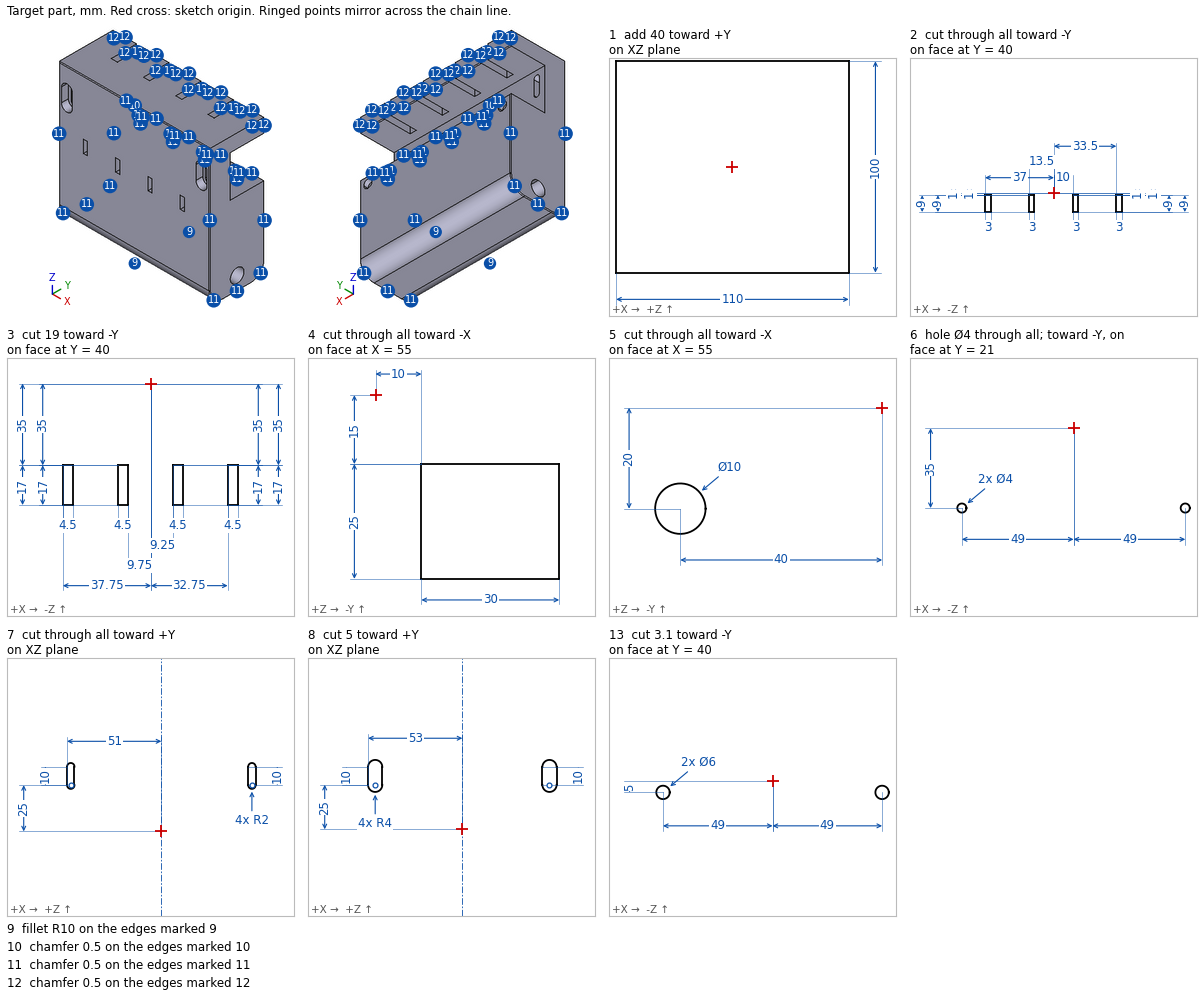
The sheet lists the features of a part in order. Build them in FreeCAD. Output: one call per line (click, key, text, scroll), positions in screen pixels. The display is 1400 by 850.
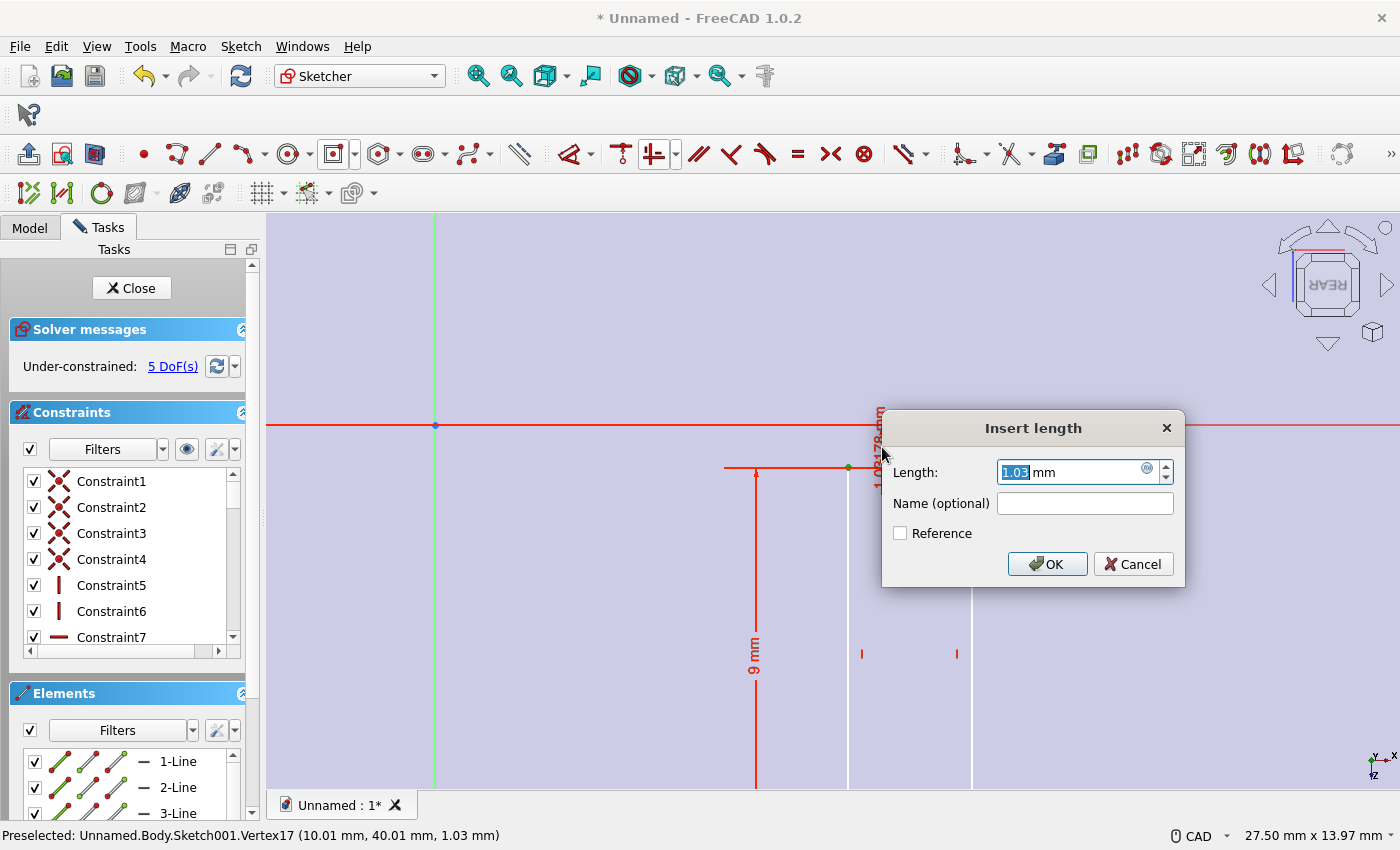
text(1)
key(Return)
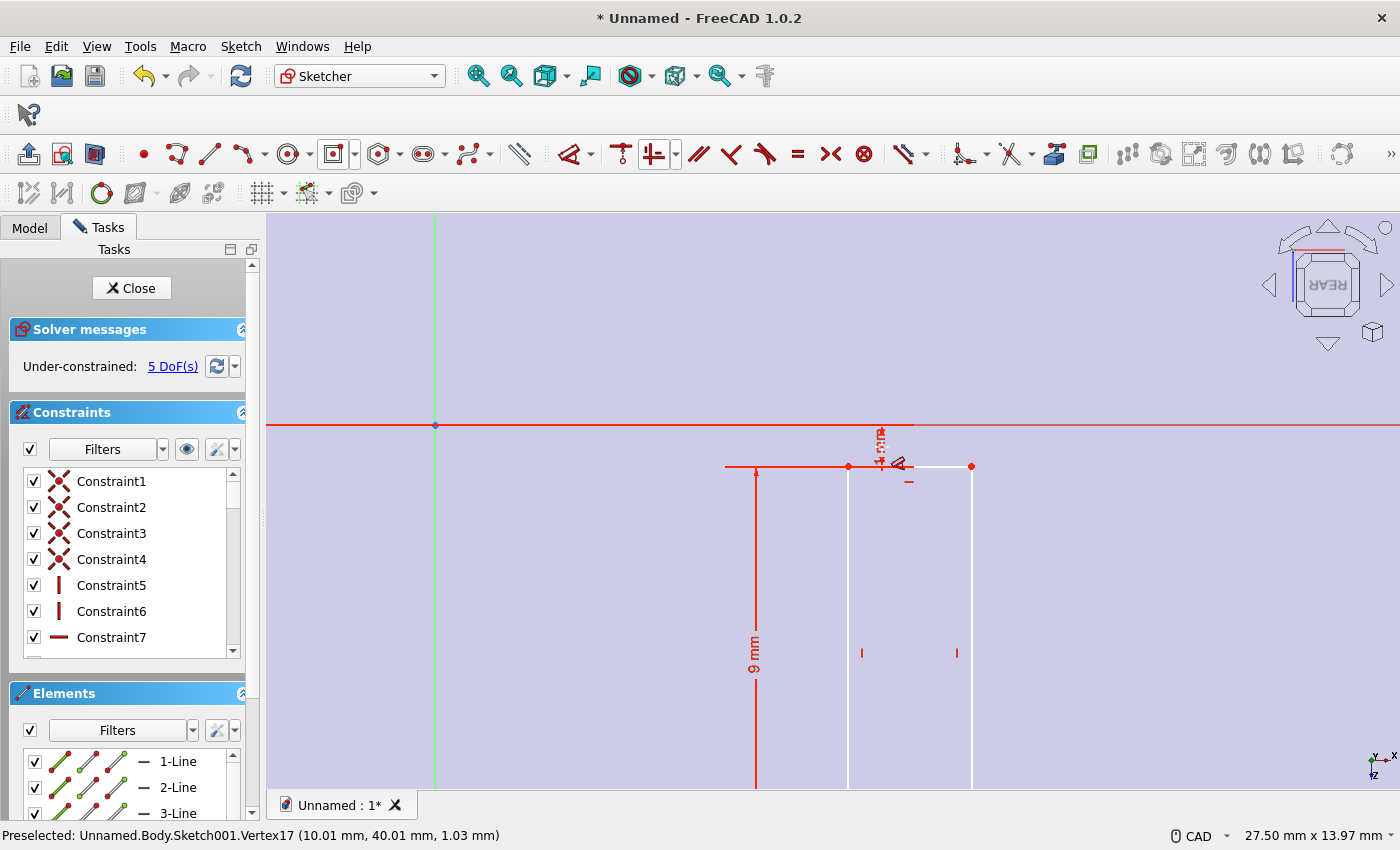
scroll(850, 468, down, 8)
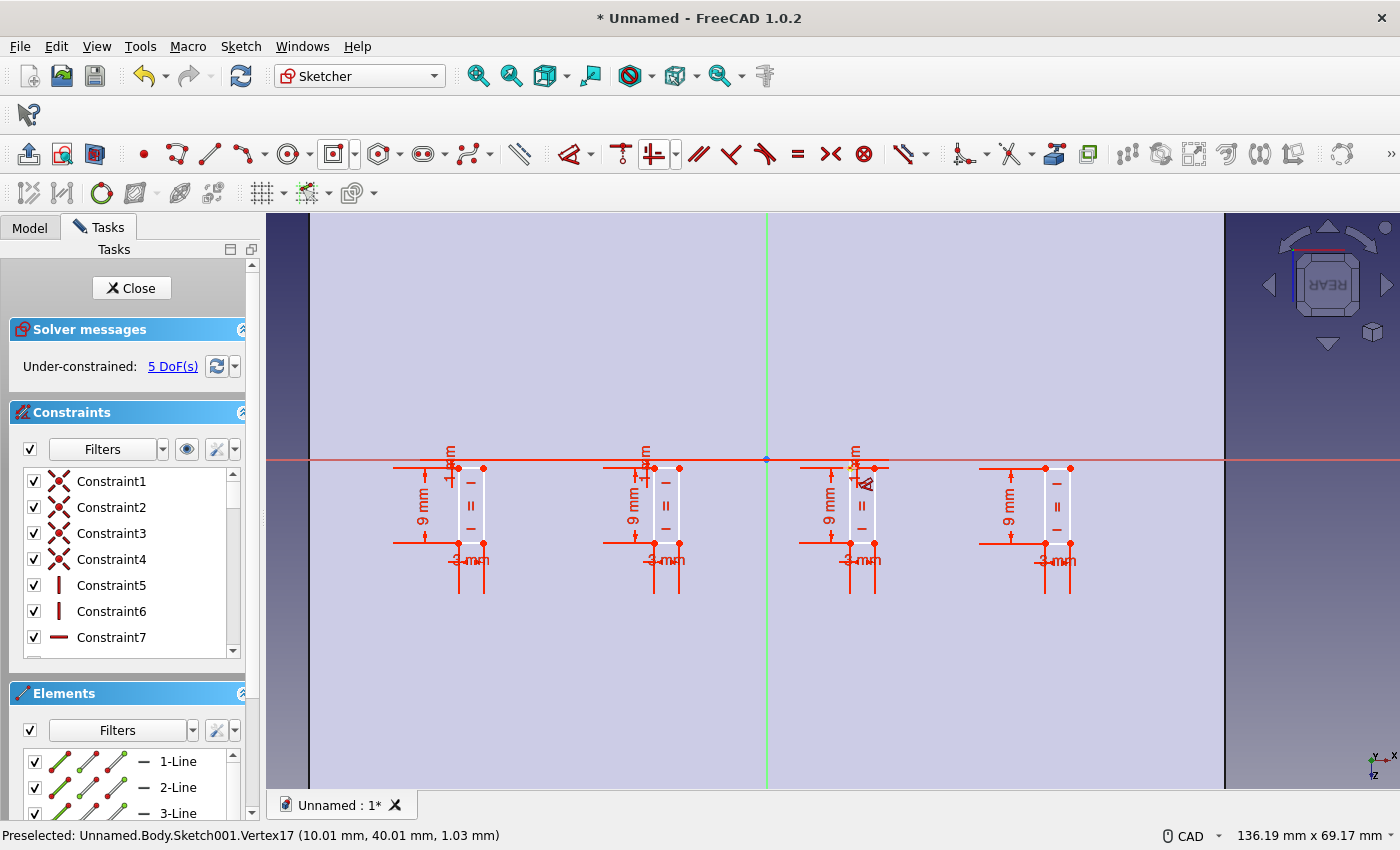
scroll(1045, 469, up, 8)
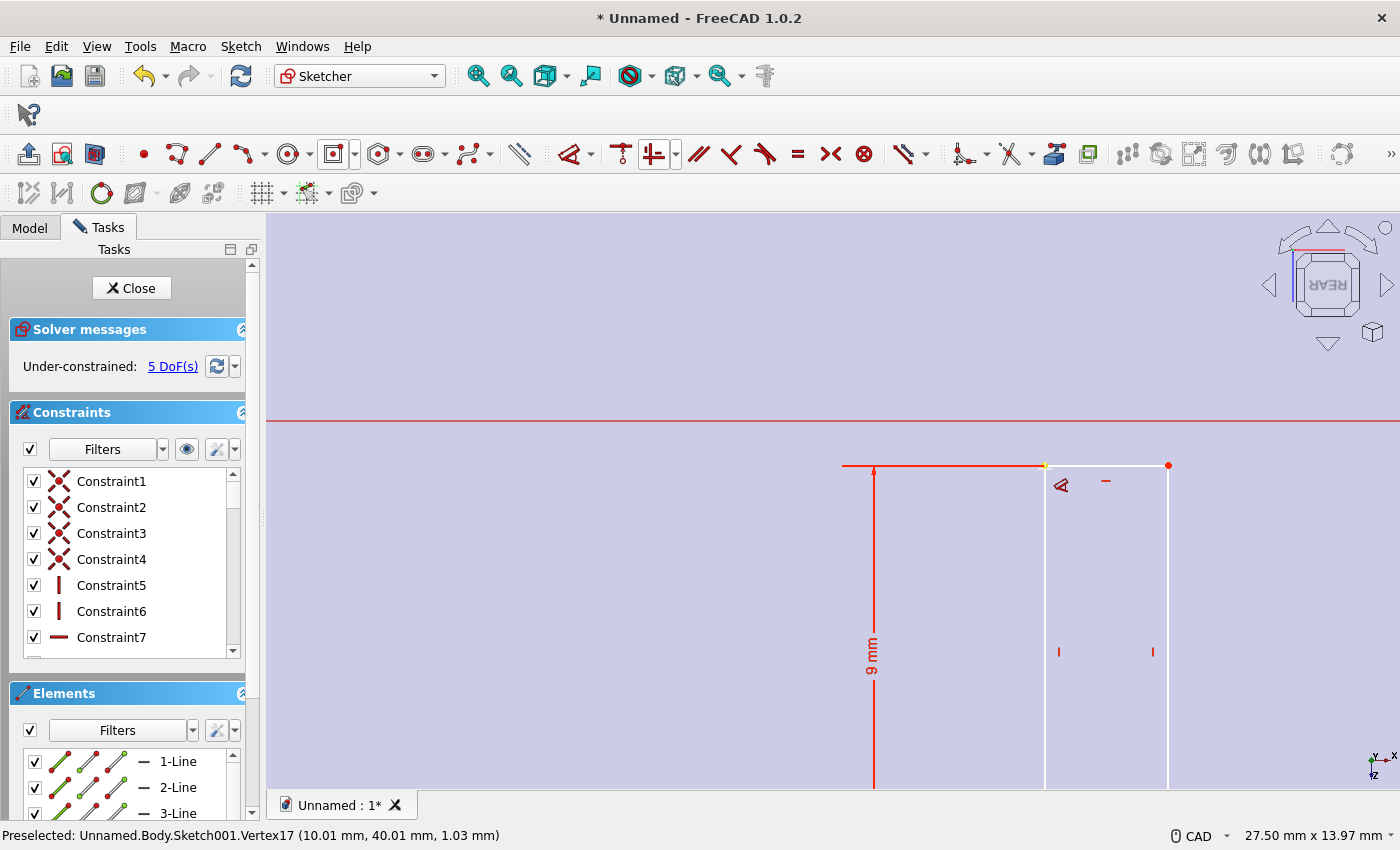
click(1045, 466)
click(1079, 444)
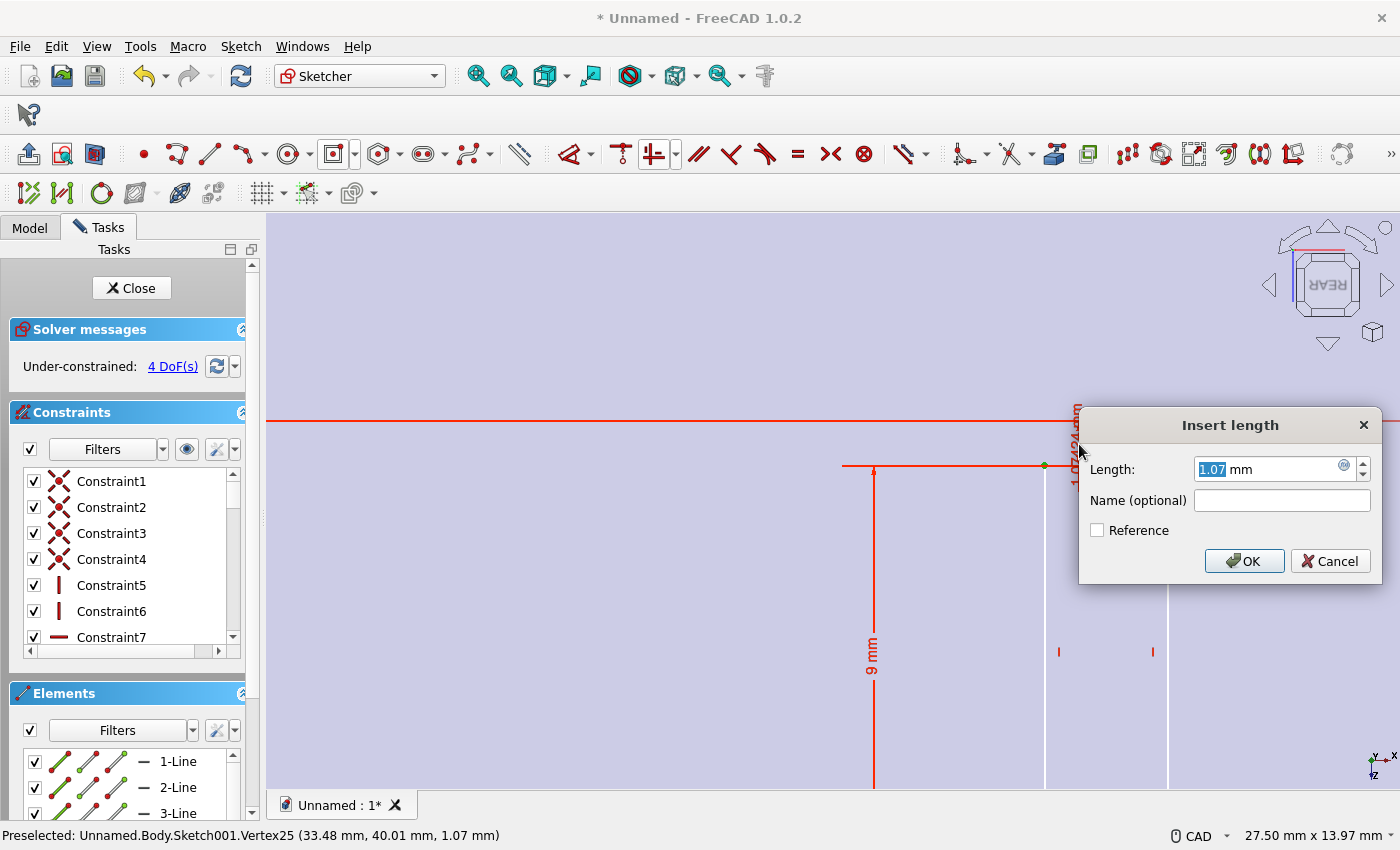
text(1)
key(Return)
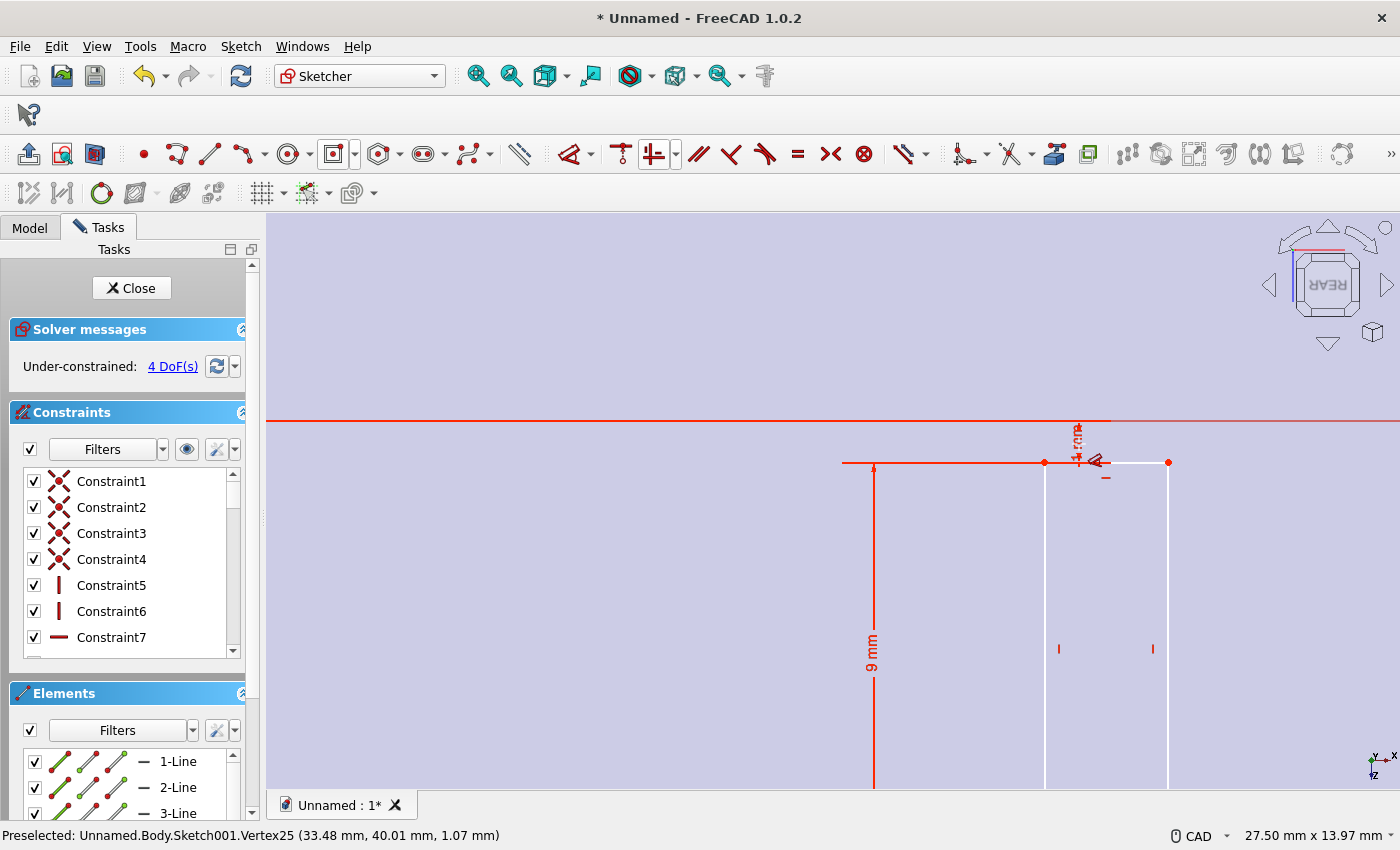
scroll(1046, 469, down, 8)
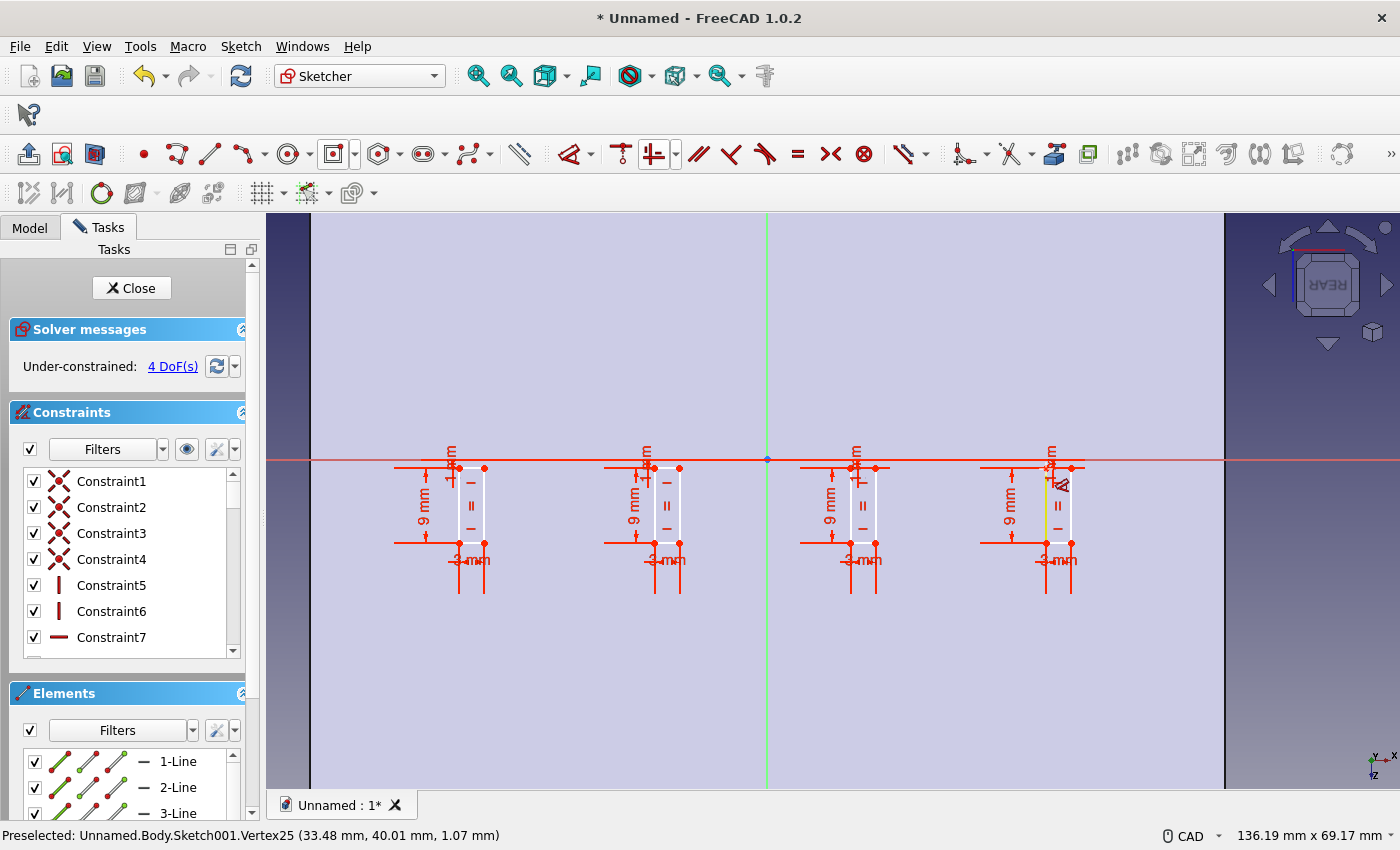
click(459, 468)
click(613, 426)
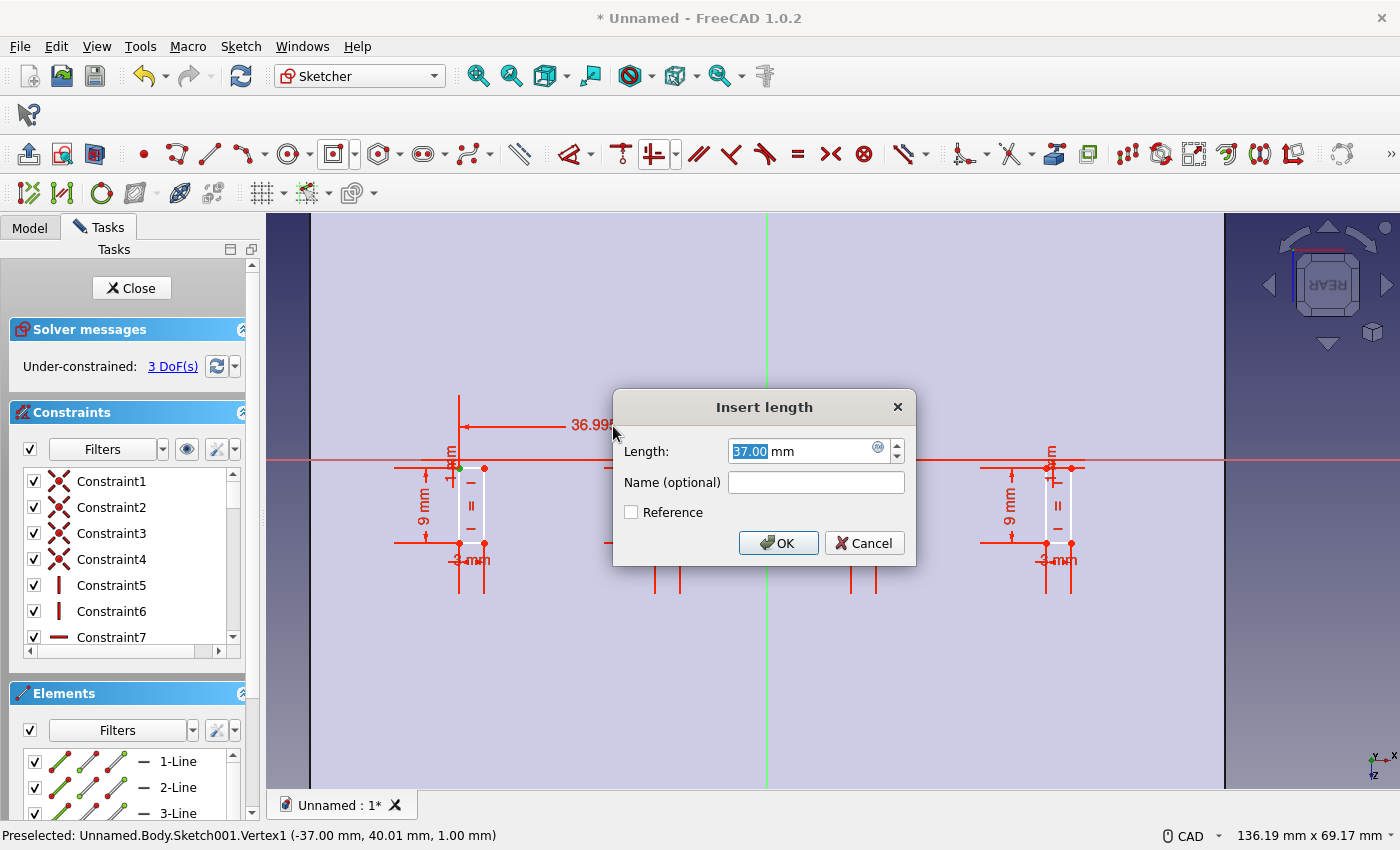
text(37)
key(Return)